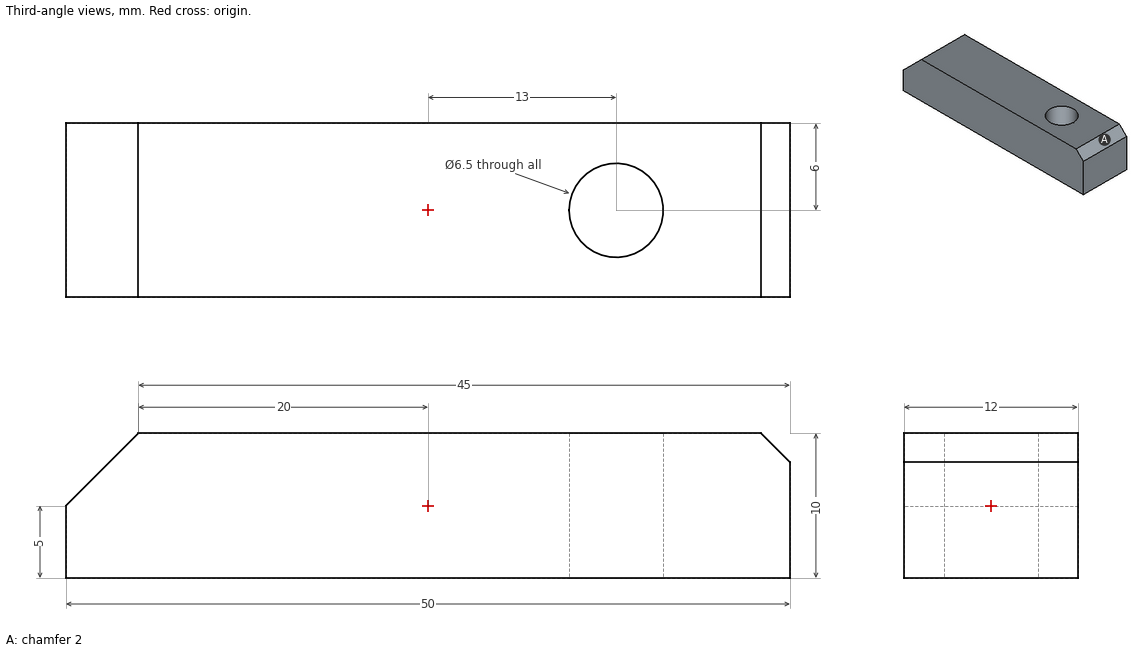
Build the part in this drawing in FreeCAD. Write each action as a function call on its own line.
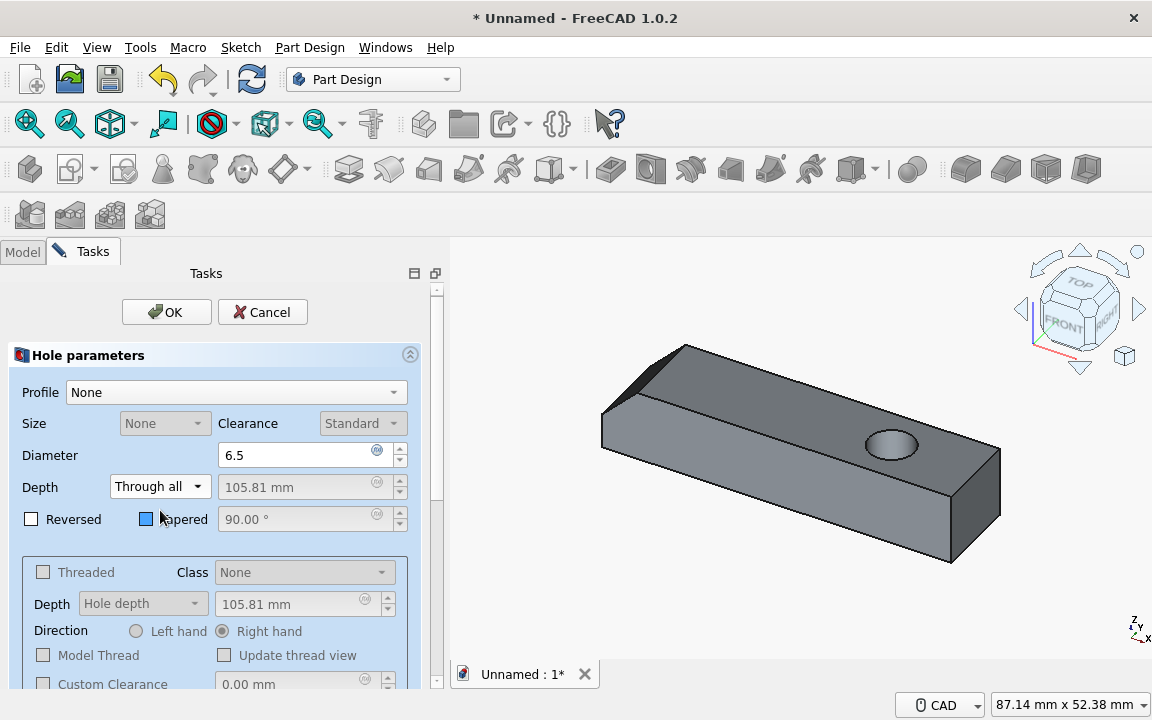
click(167, 312)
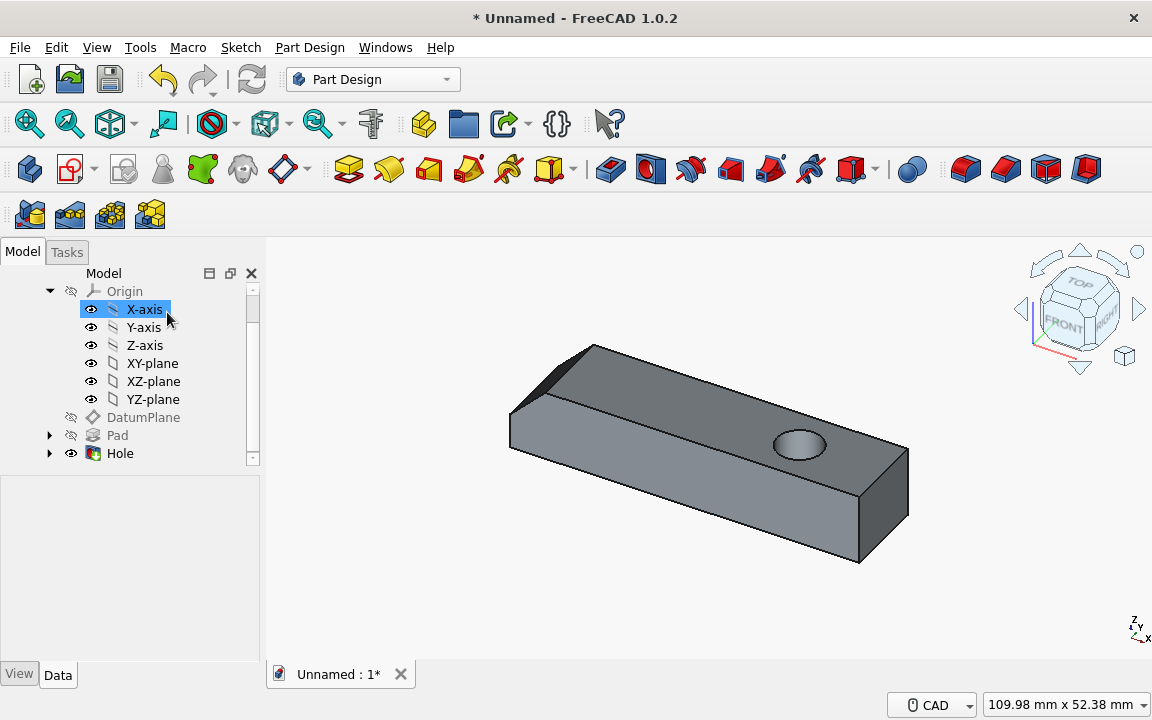
click(883, 472)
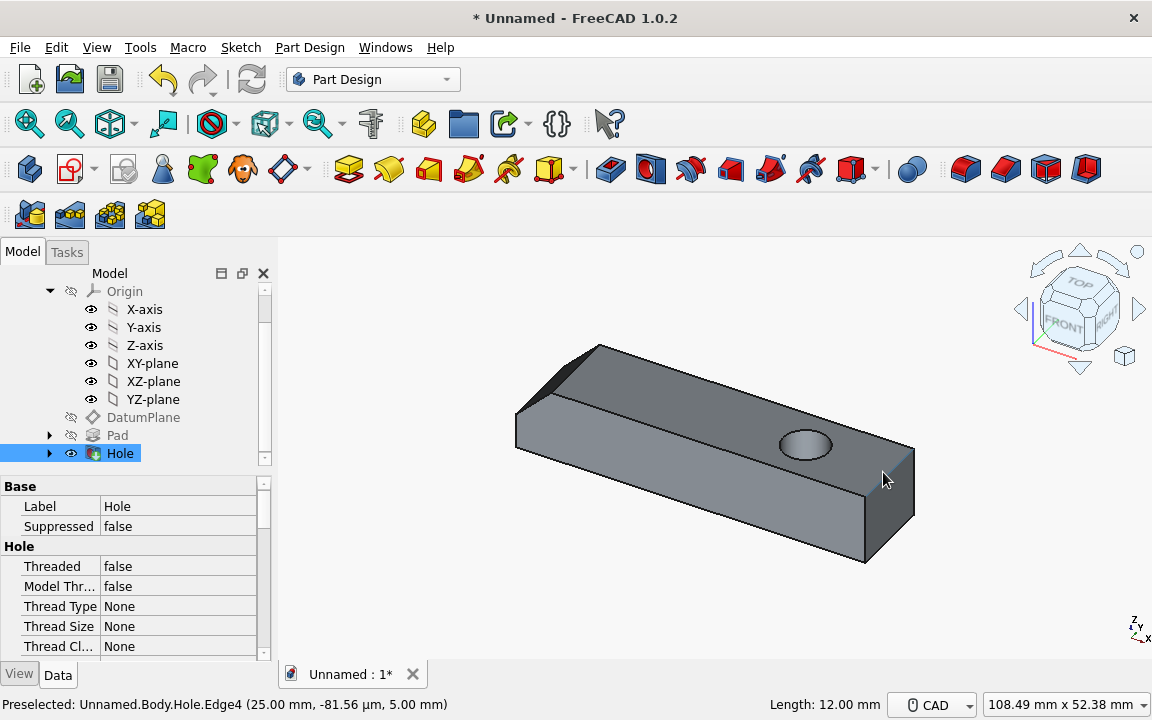
click(1006, 170)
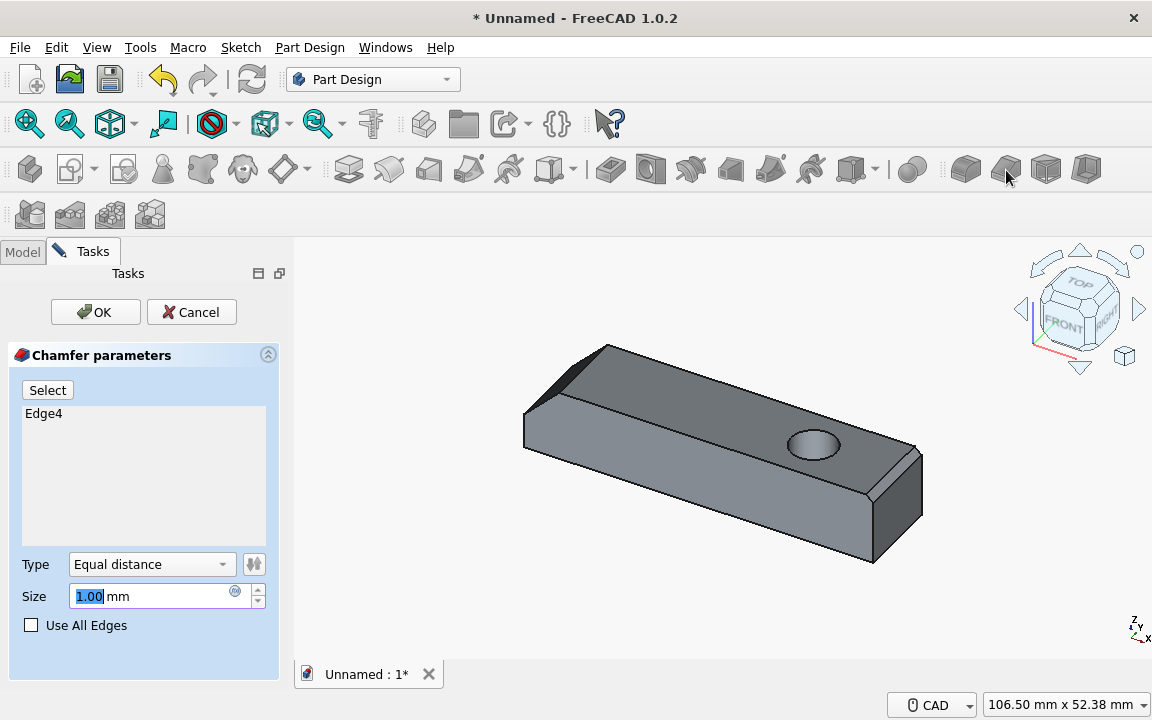
text(2)
key(Tab)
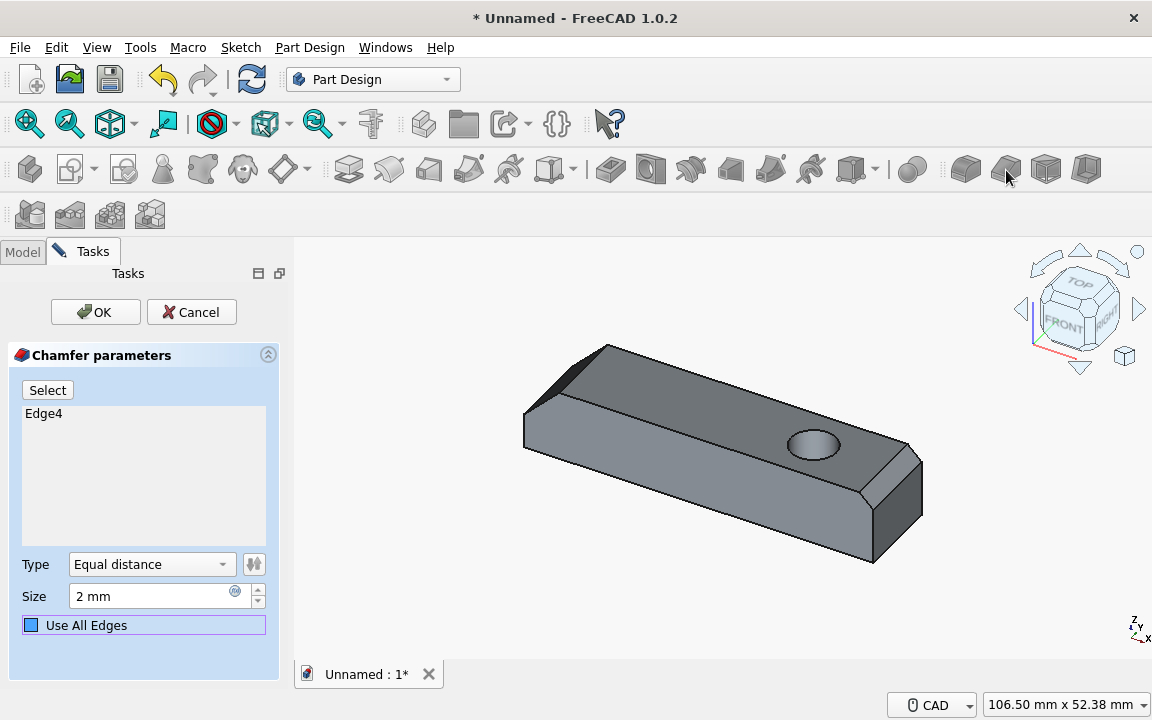
click(96, 312)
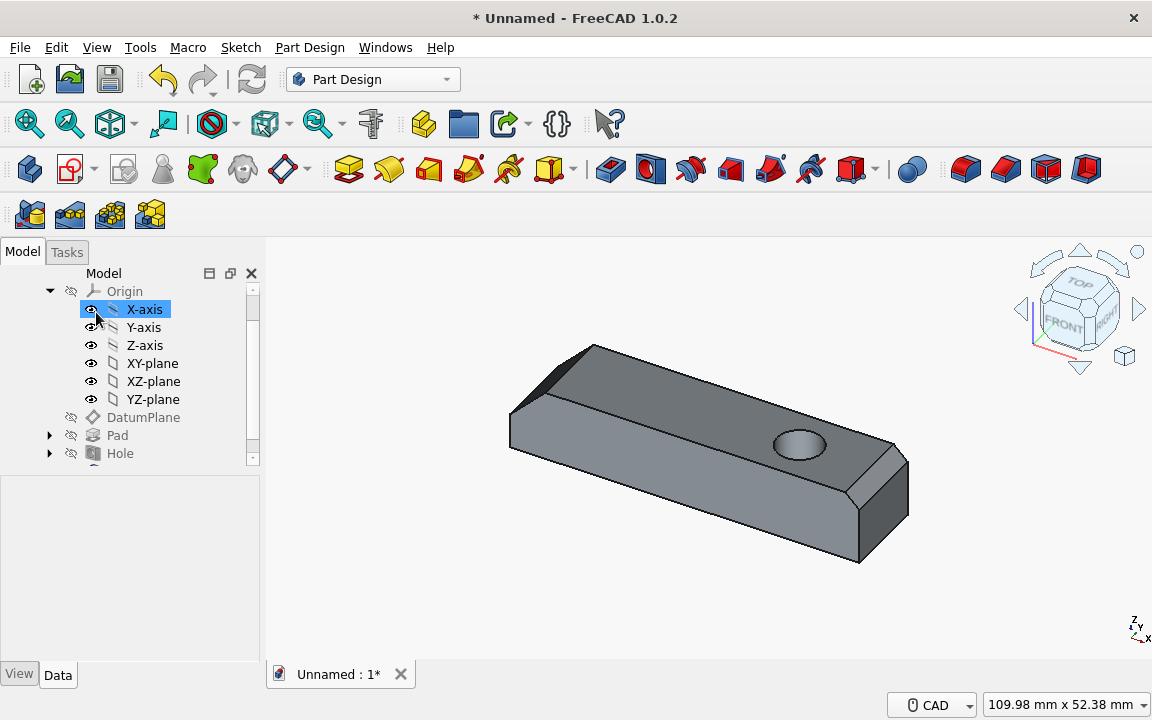
key(0)